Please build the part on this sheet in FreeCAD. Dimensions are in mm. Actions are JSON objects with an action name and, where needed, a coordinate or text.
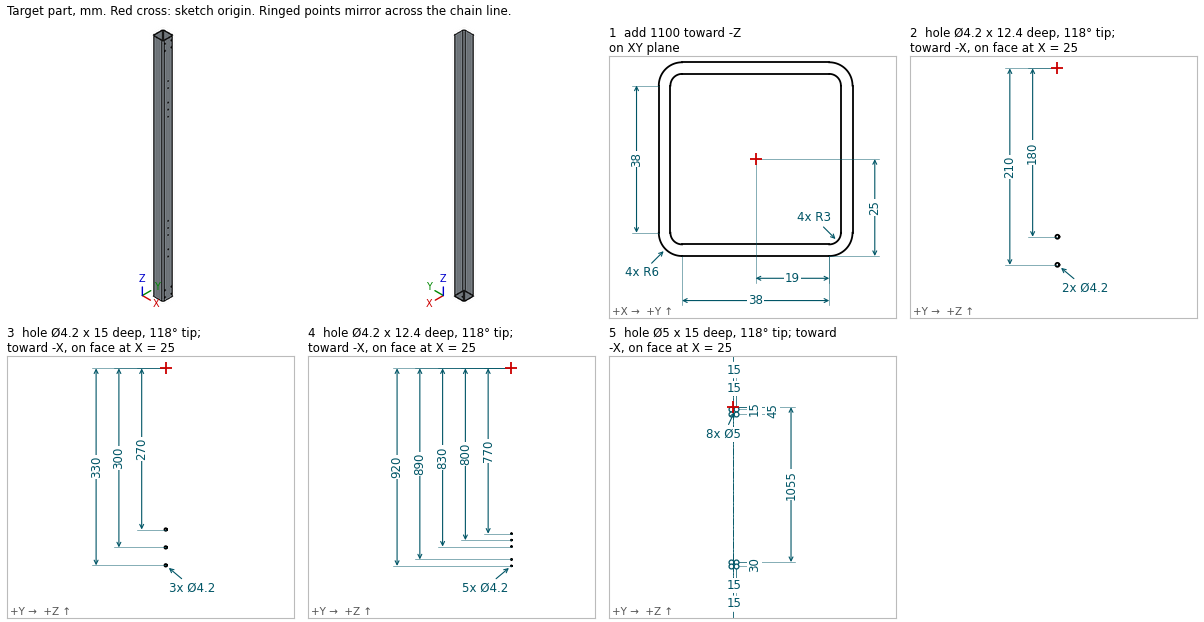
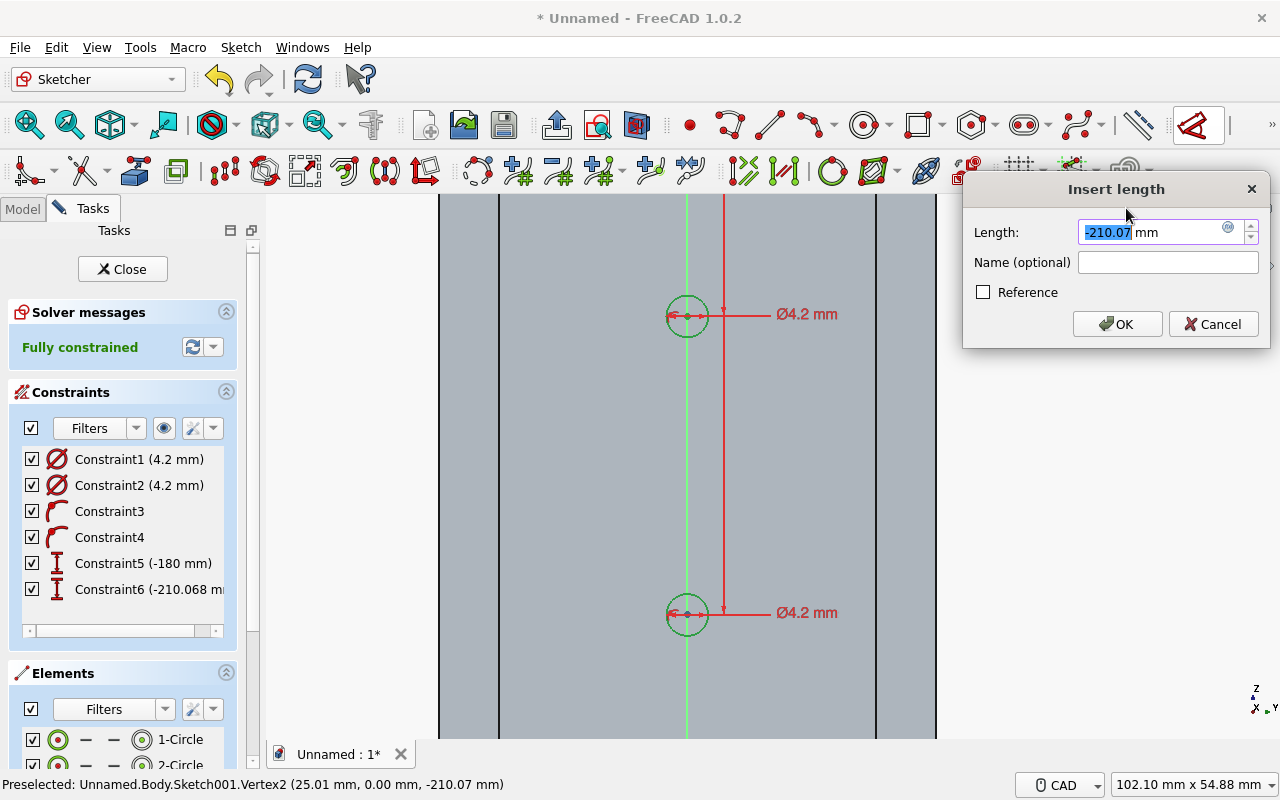
{"action": "type", "text": "-210"}
{"action": "key", "text": "Return"}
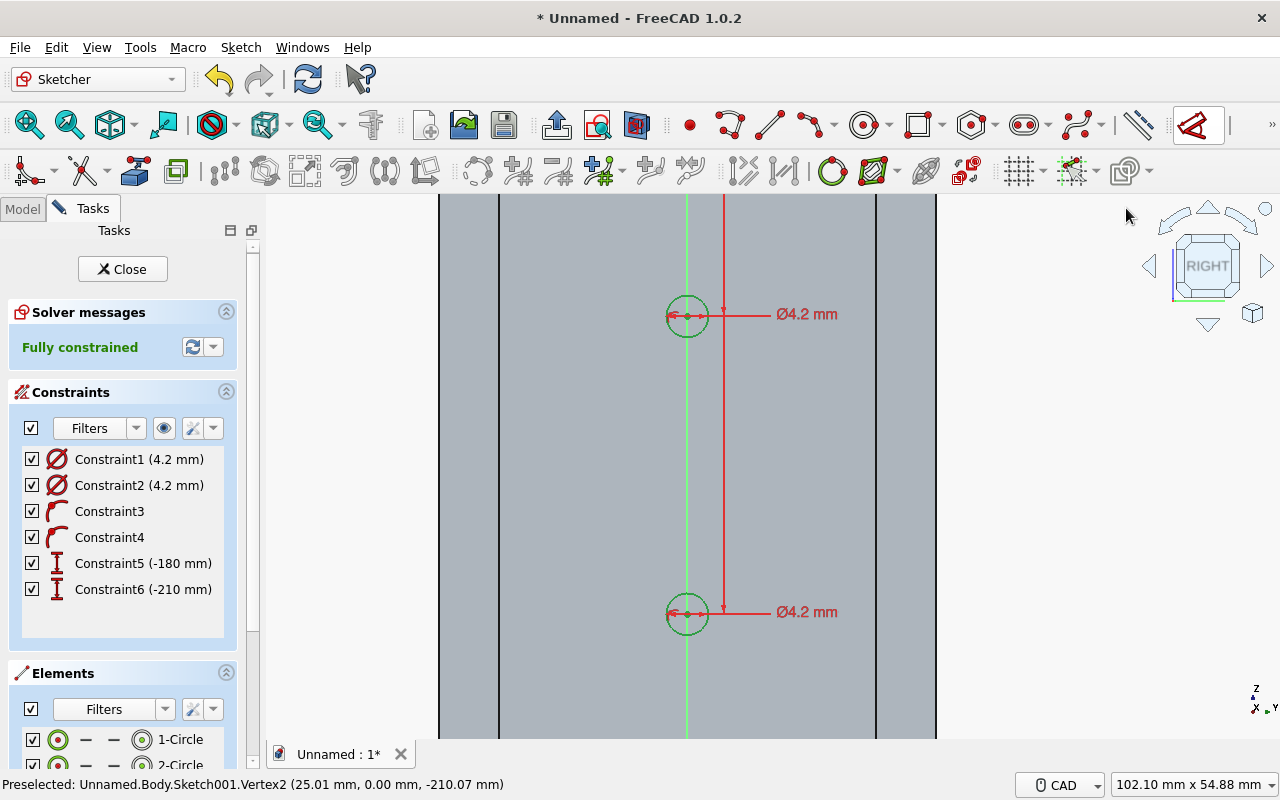
{"action": "left_click", "coordinate": [123, 269]}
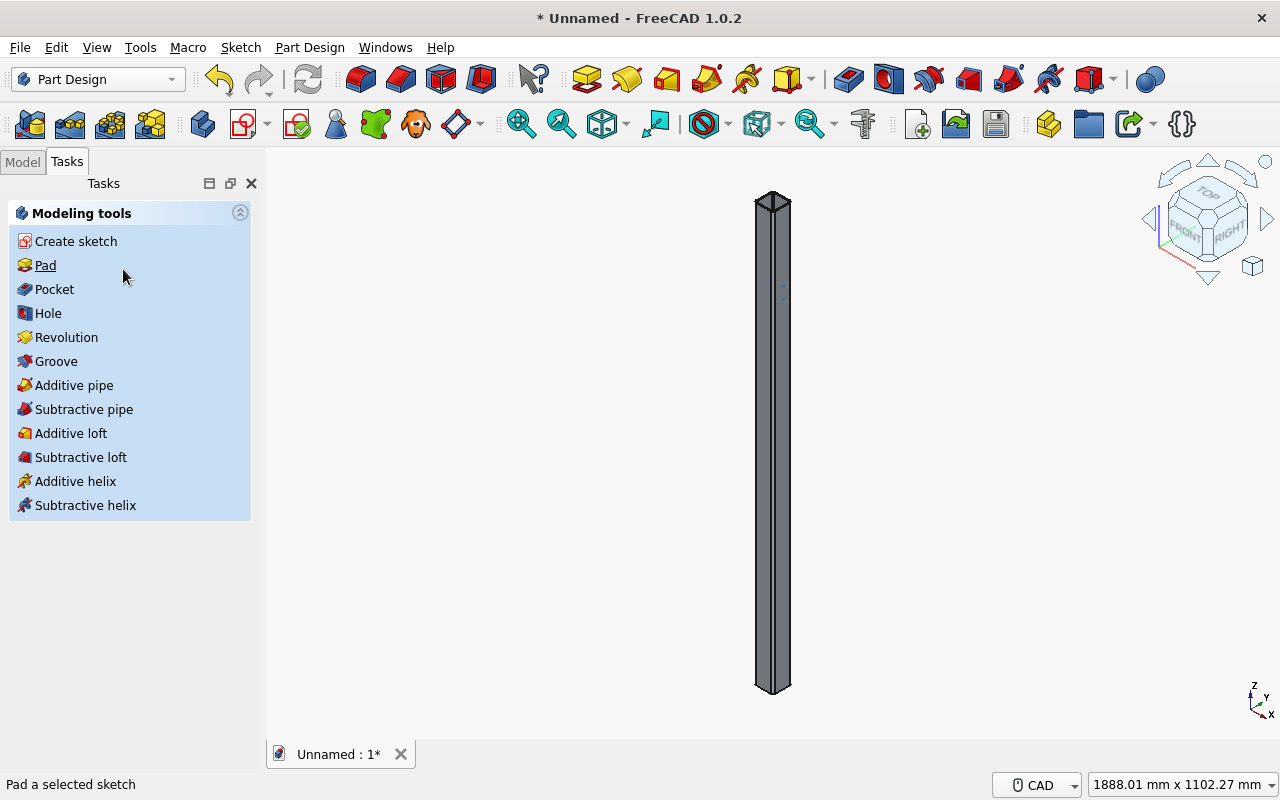
{"action": "left_click", "coordinate": [890, 80]}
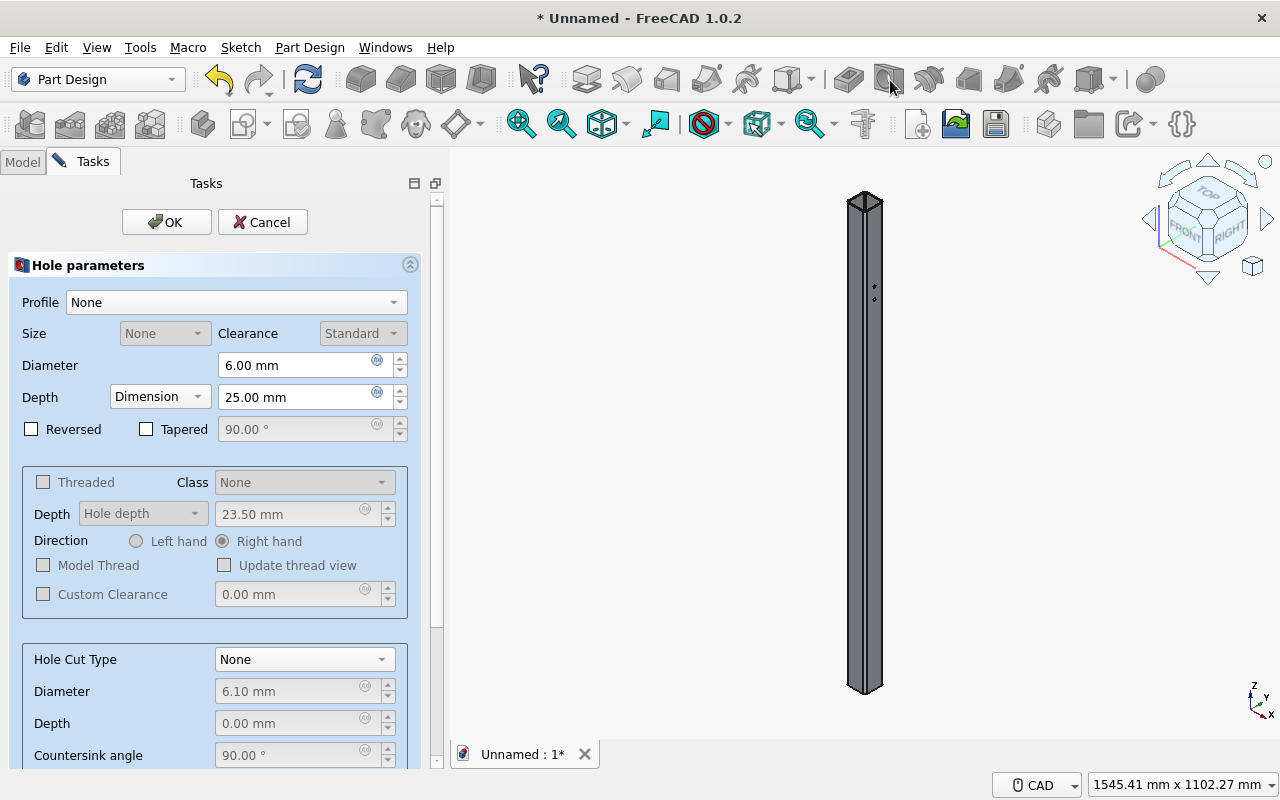
{"action": "triple_click", "coordinate": [305, 365]}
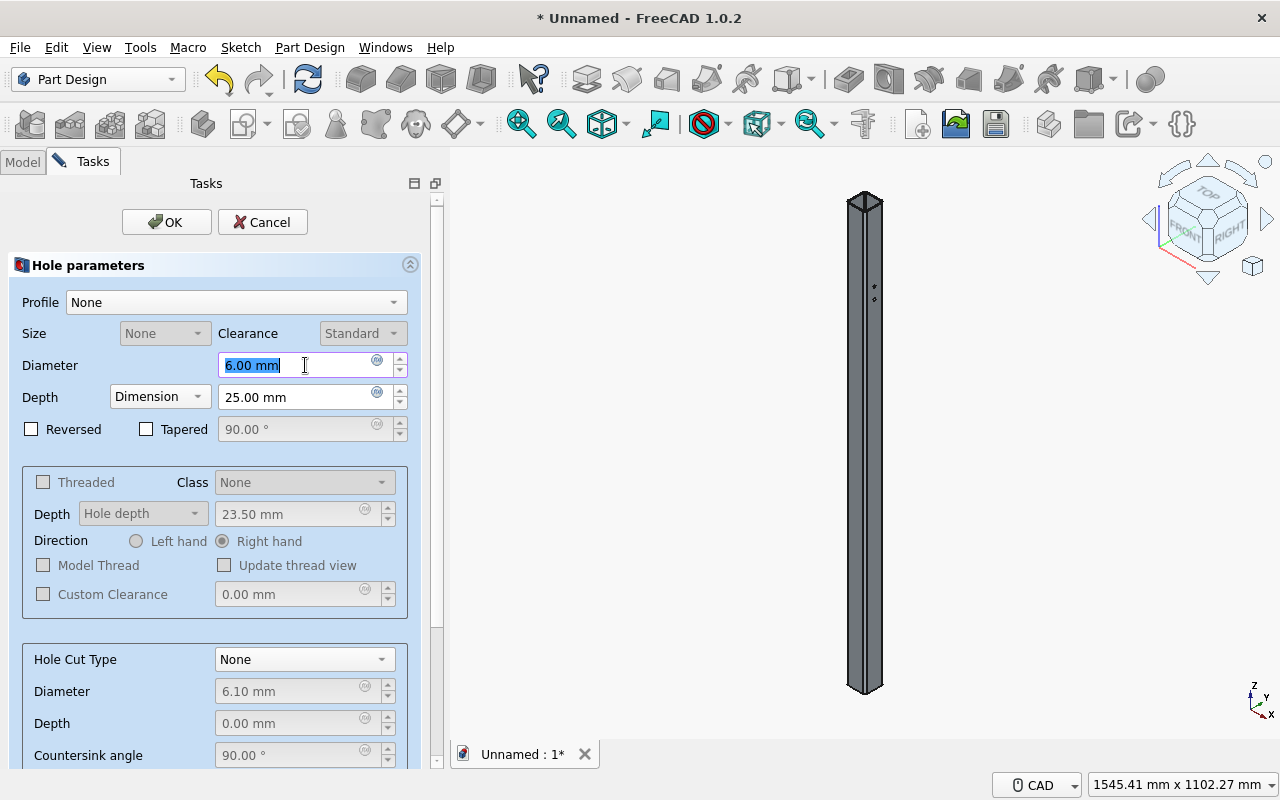
{"action": "type", "text": "4.2"}
{"action": "key", "text": "Tab"}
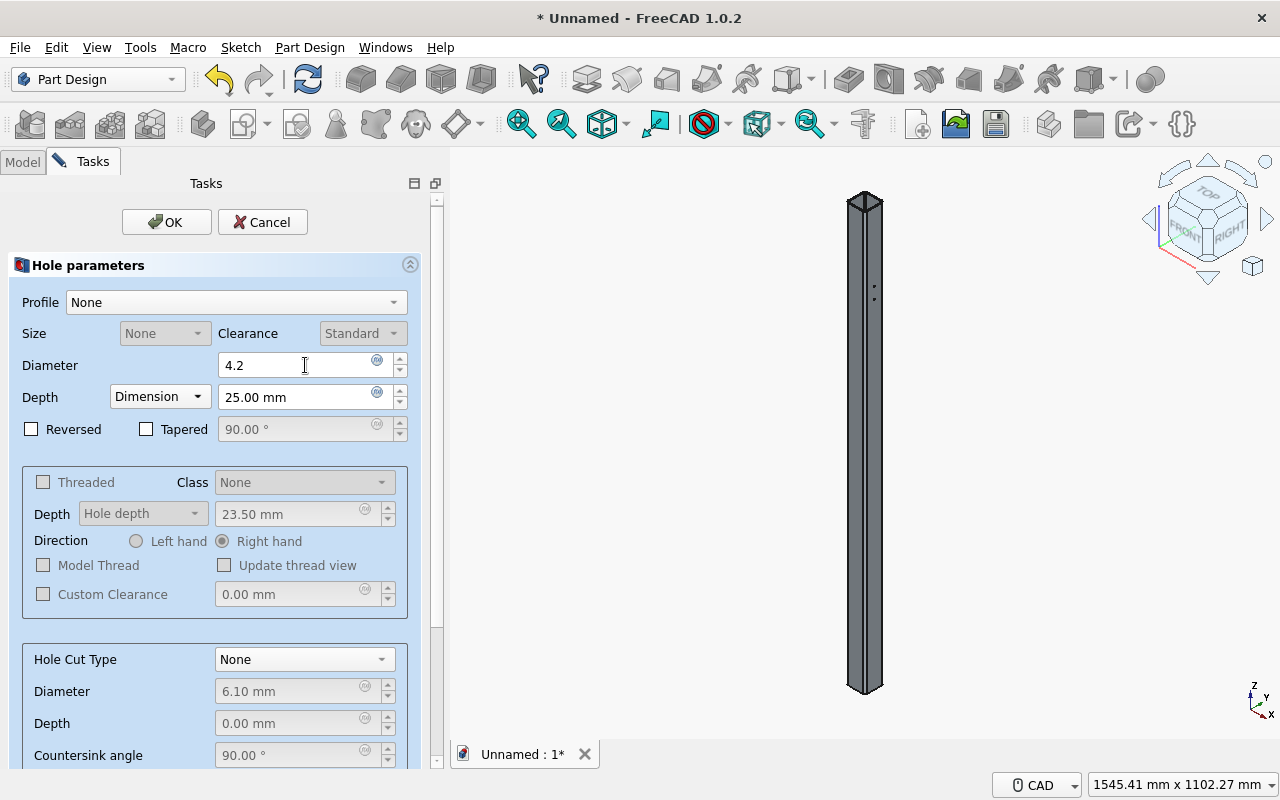
{"action": "triple_click", "coordinate": [305, 397]}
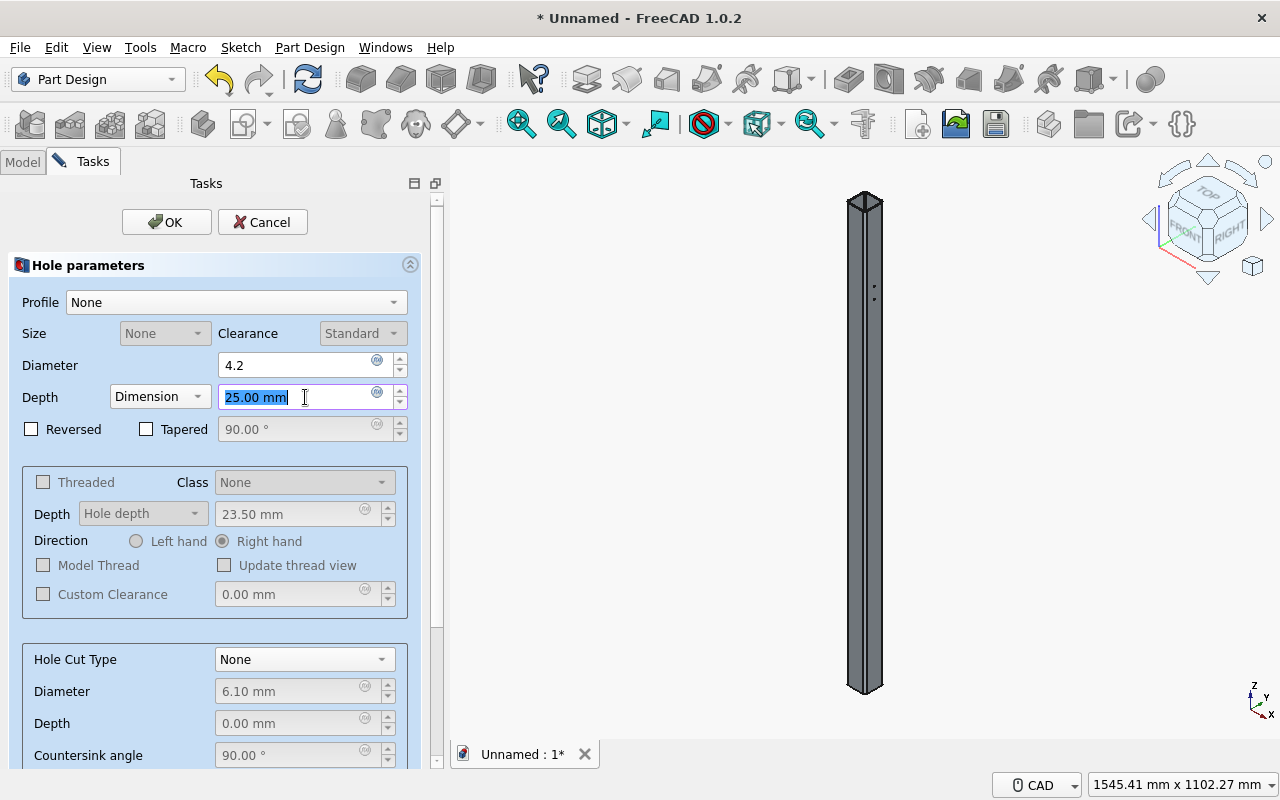
{"action": "type", "text": "12.4"}
{"action": "key", "text": "Tab"}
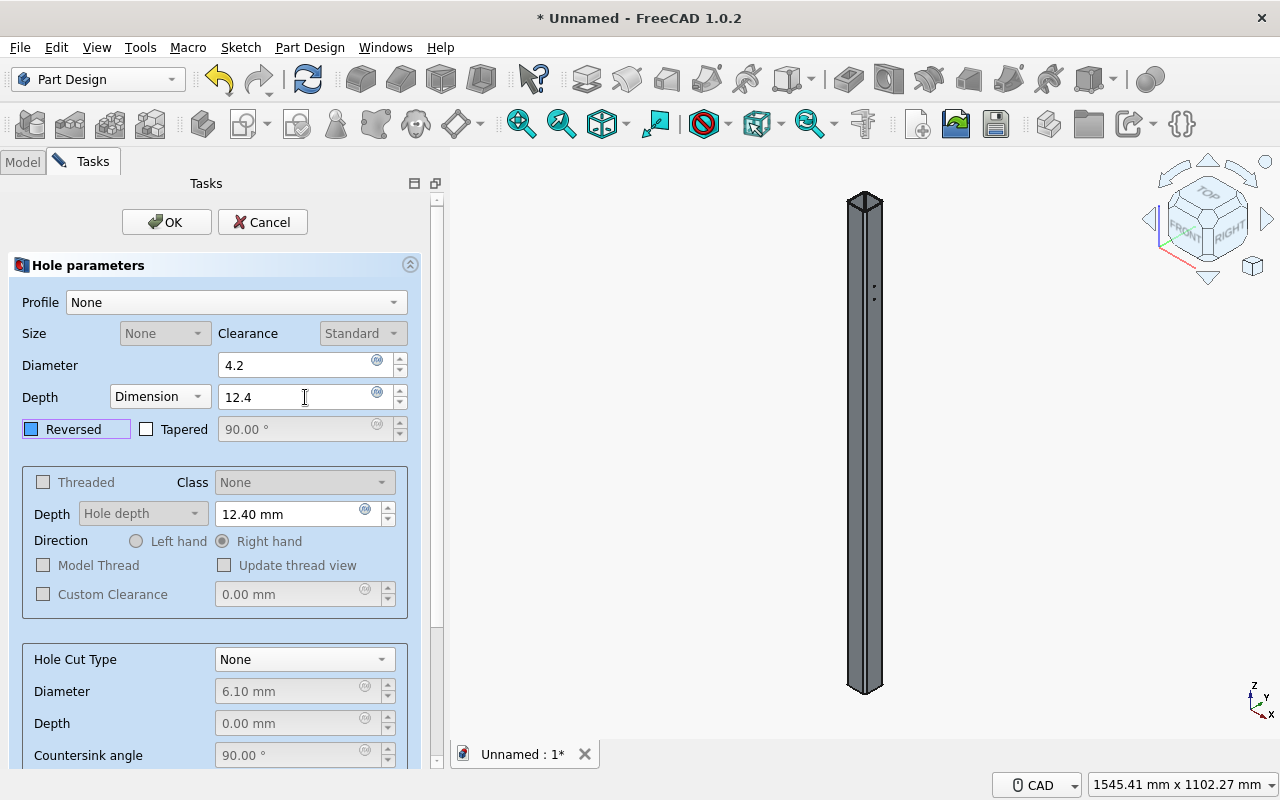
{"action": "left_click", "coordinate": [167, 222]}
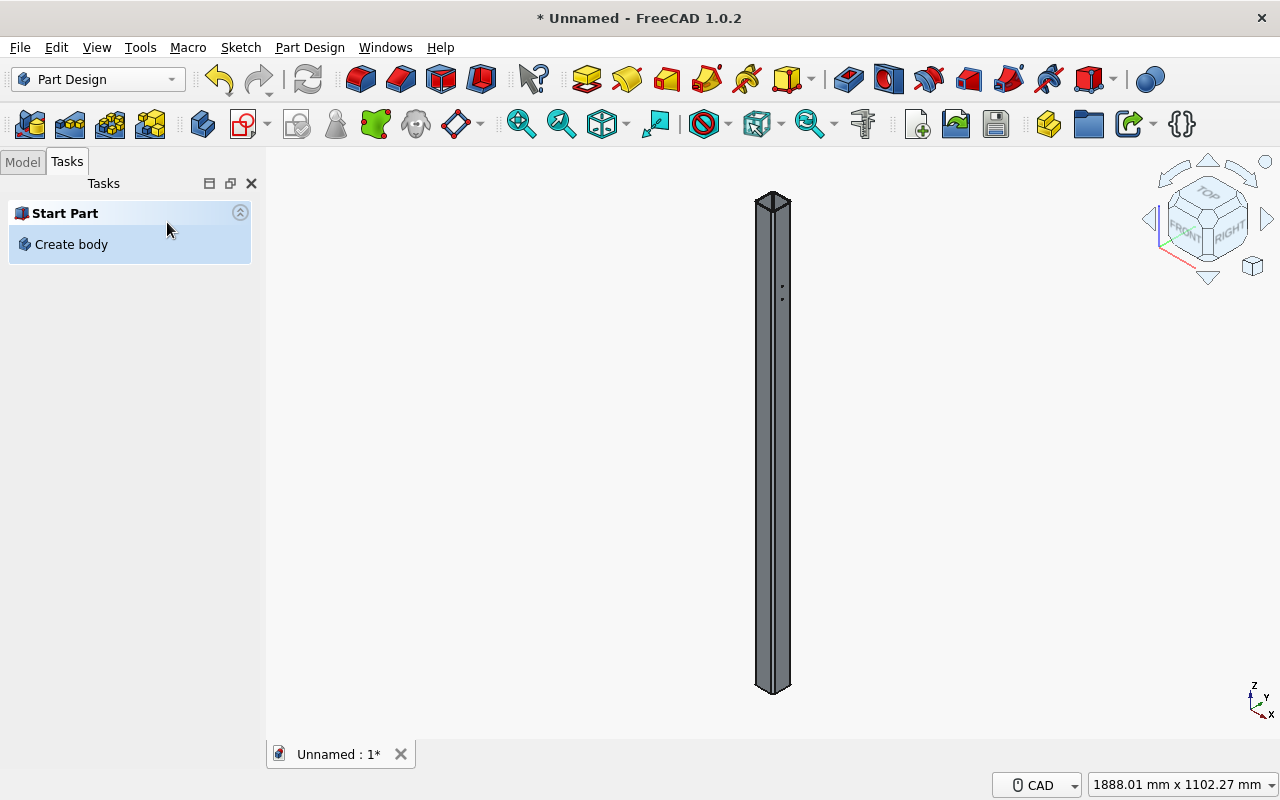
{"action": "left_click", "coordinate": [785, 240]}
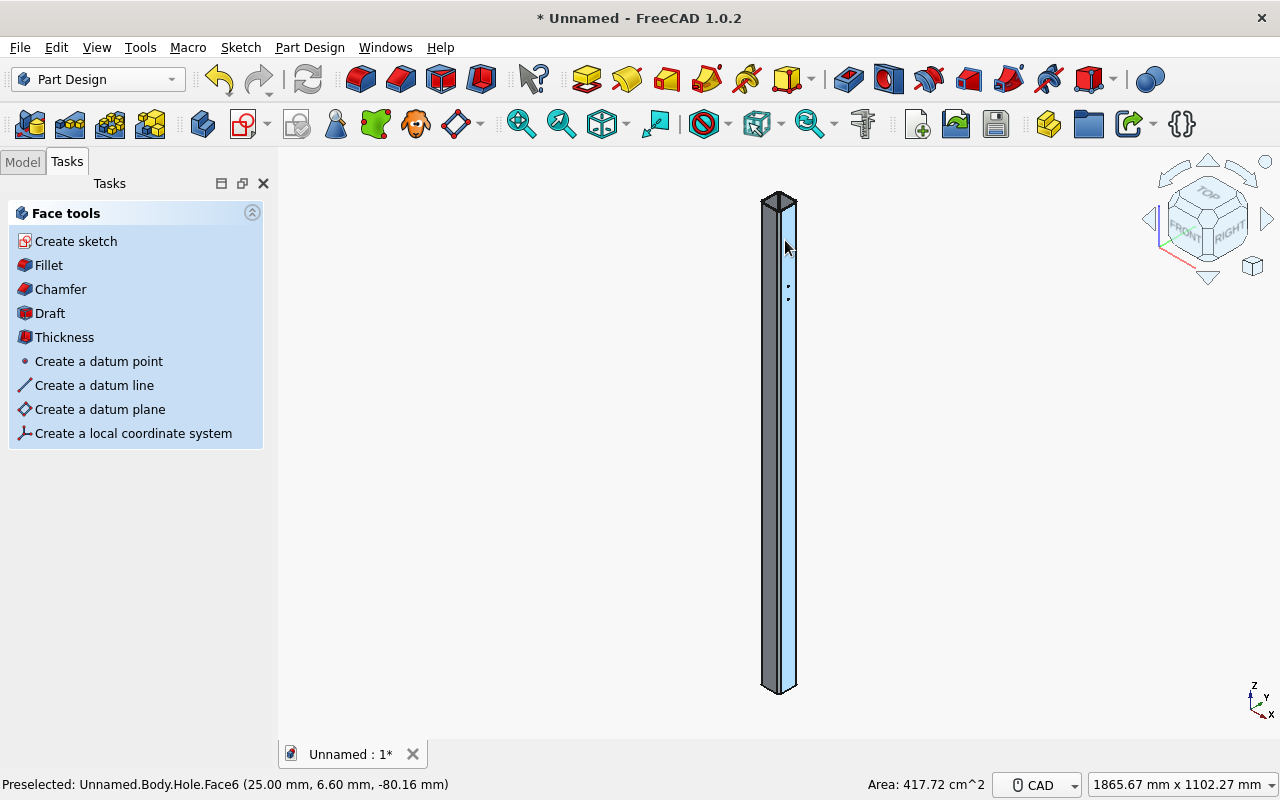
{"action": "left_click", "coordinate": [244, 124]}